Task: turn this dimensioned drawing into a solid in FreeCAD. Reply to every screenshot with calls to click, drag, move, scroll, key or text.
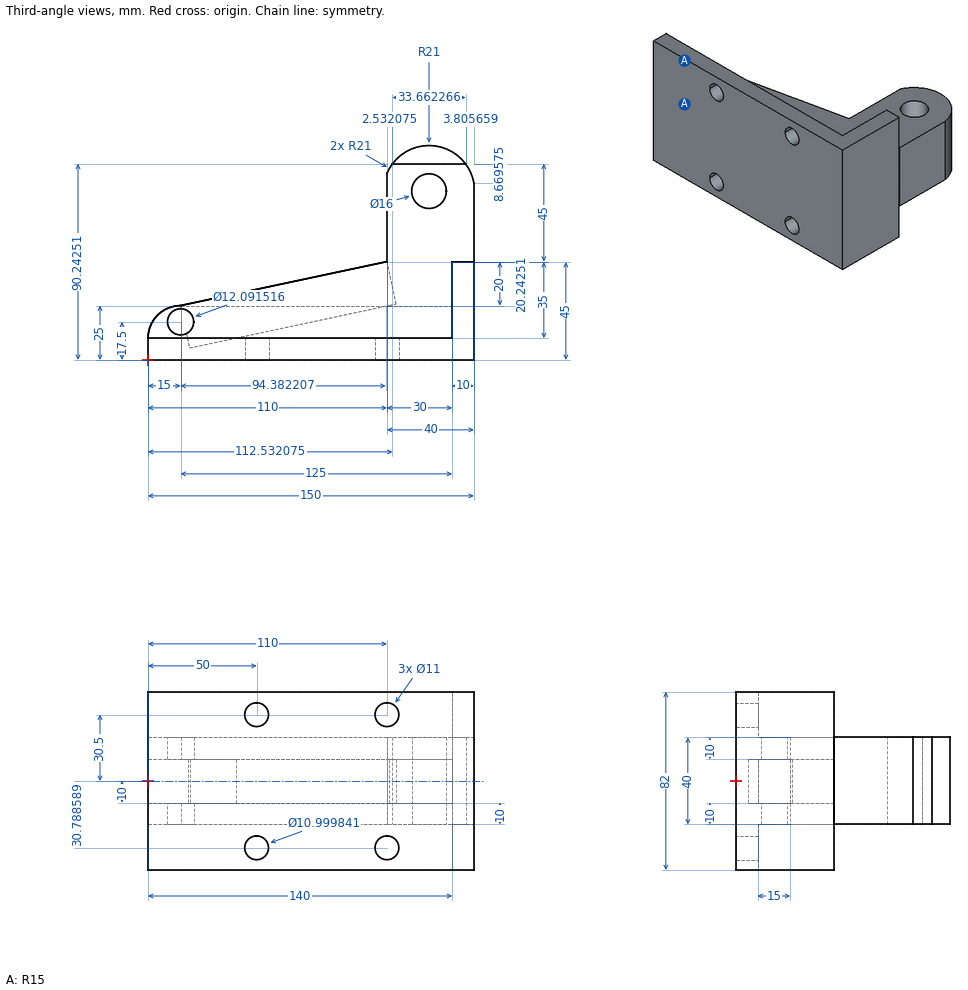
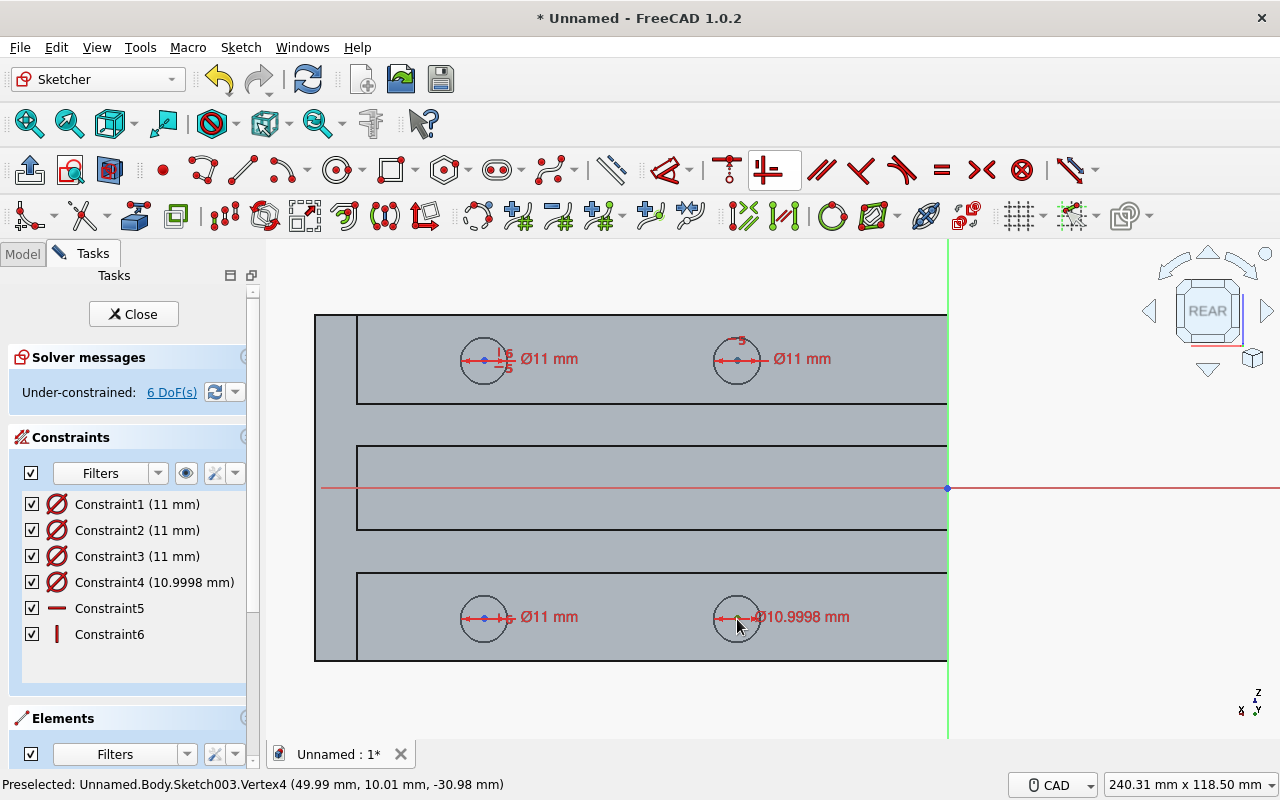
click(796, 170)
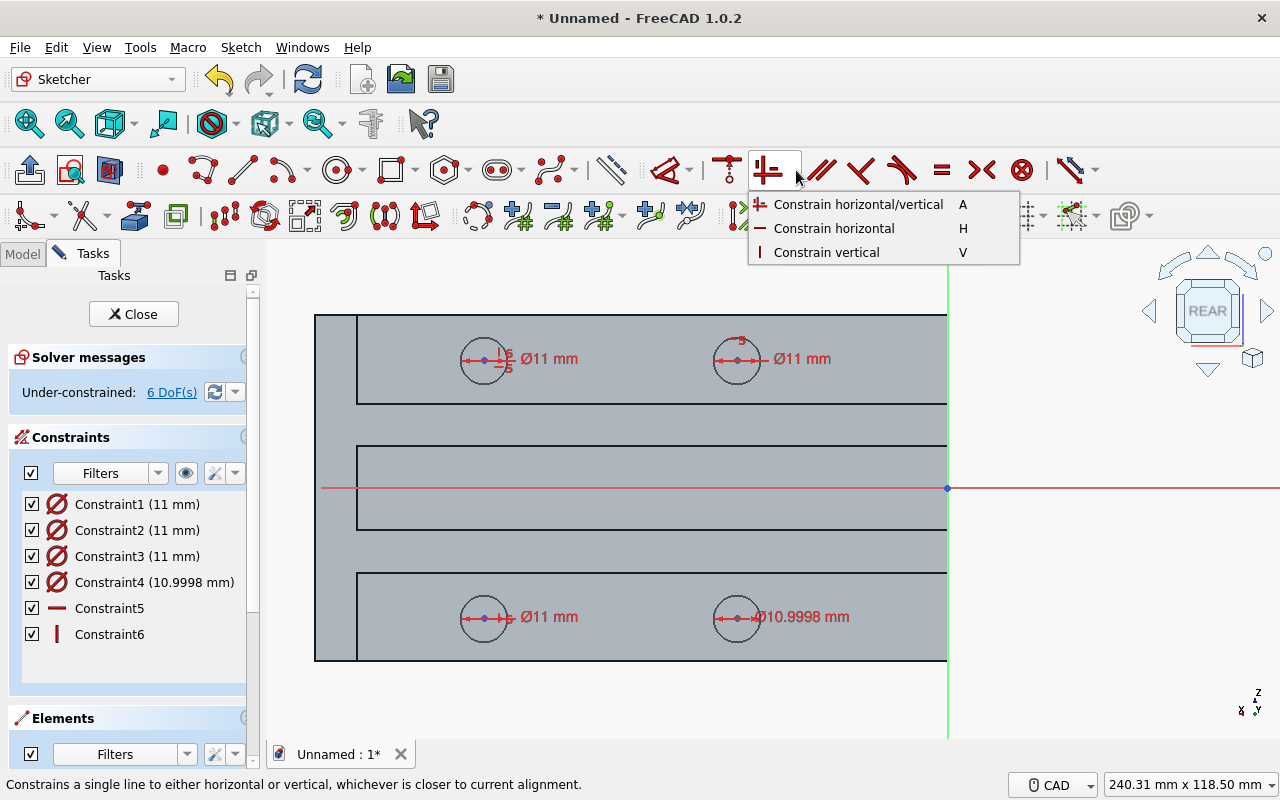
click(884, 252)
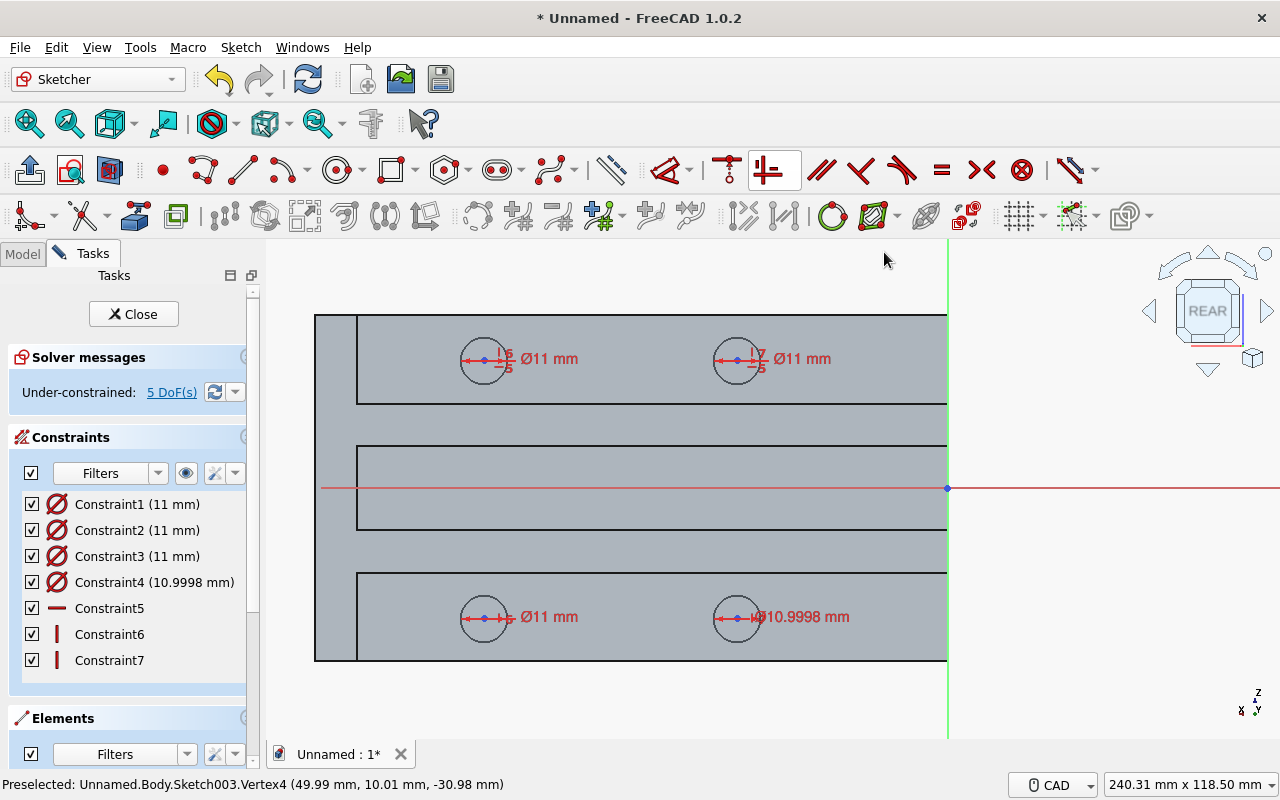
click(484, 619)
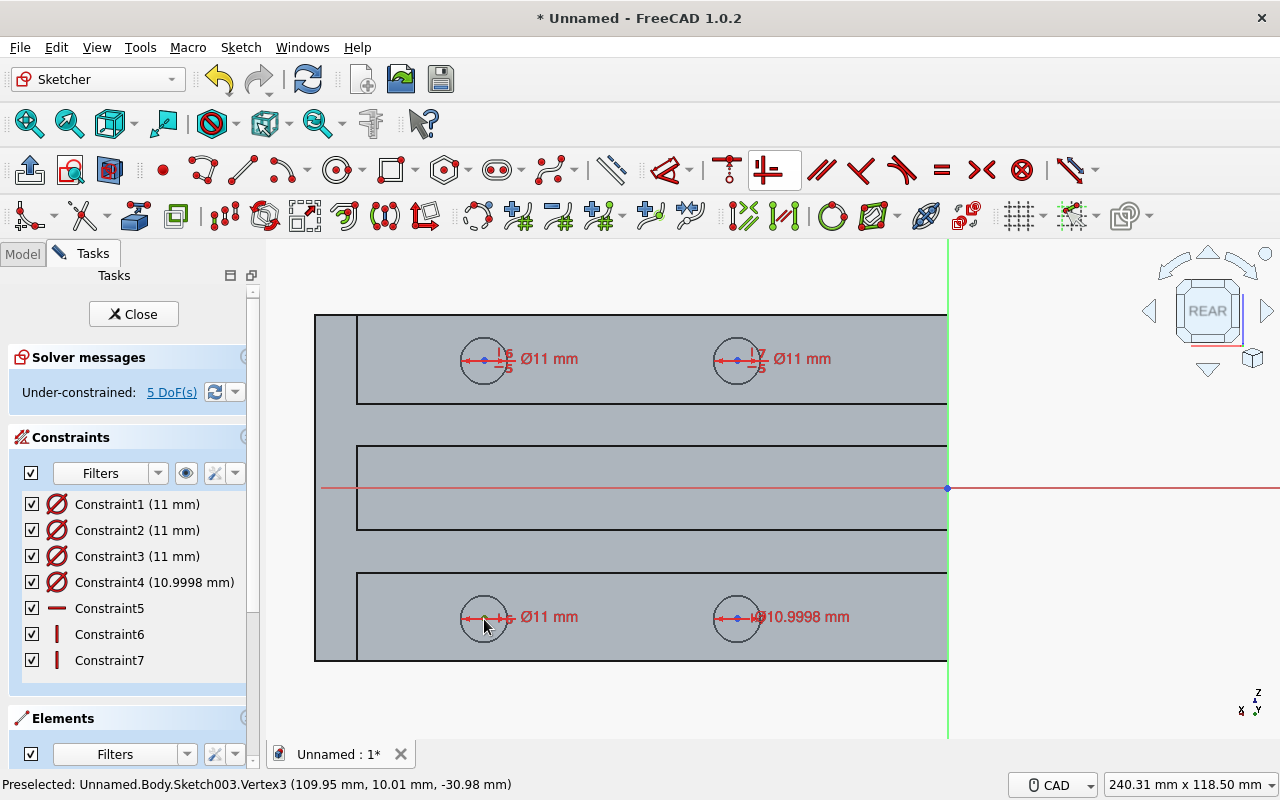
click(737, 619)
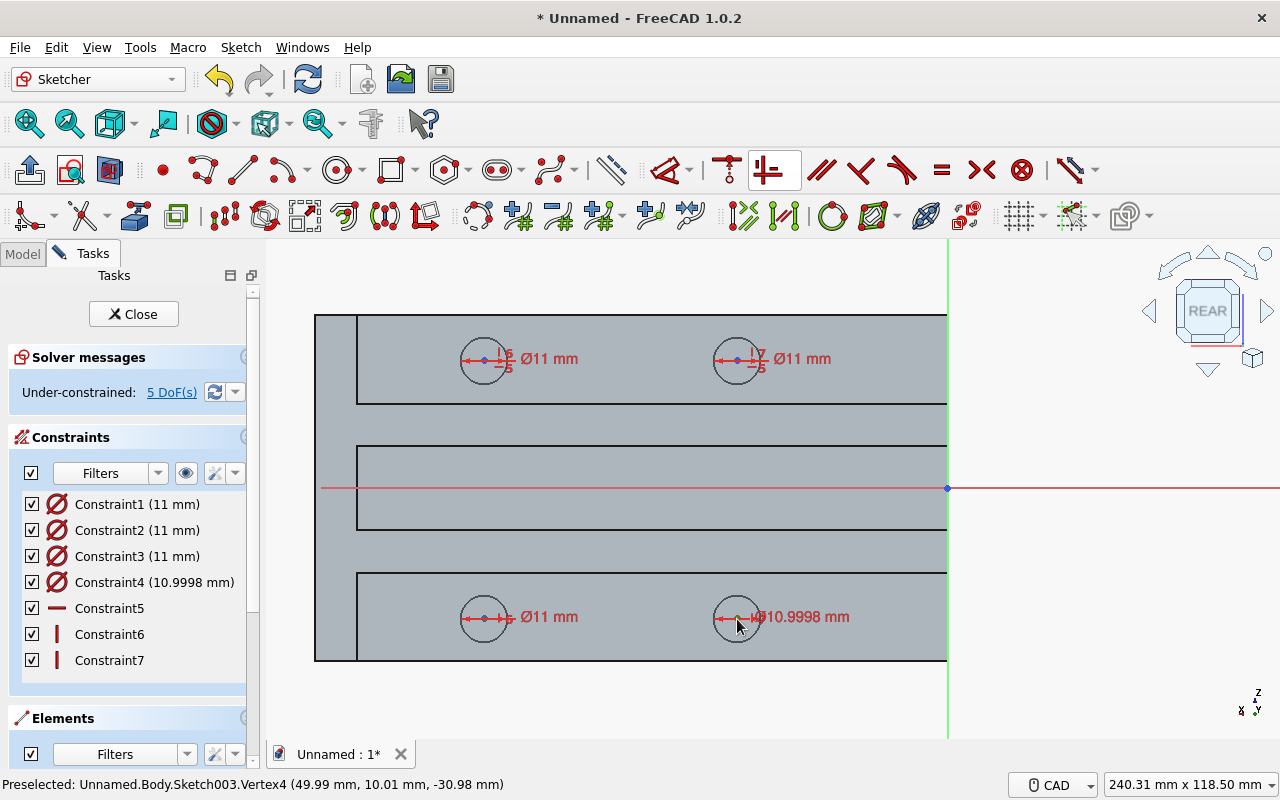
key(h)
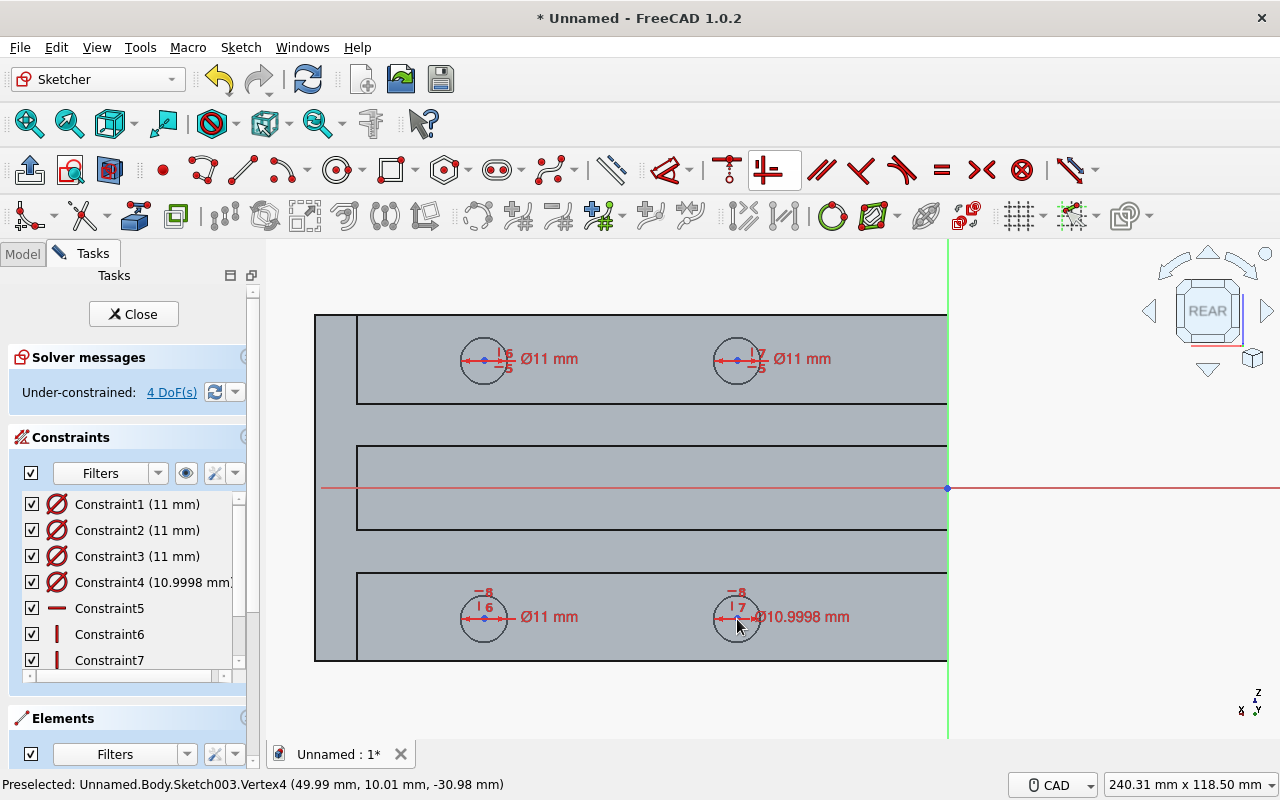
key(d)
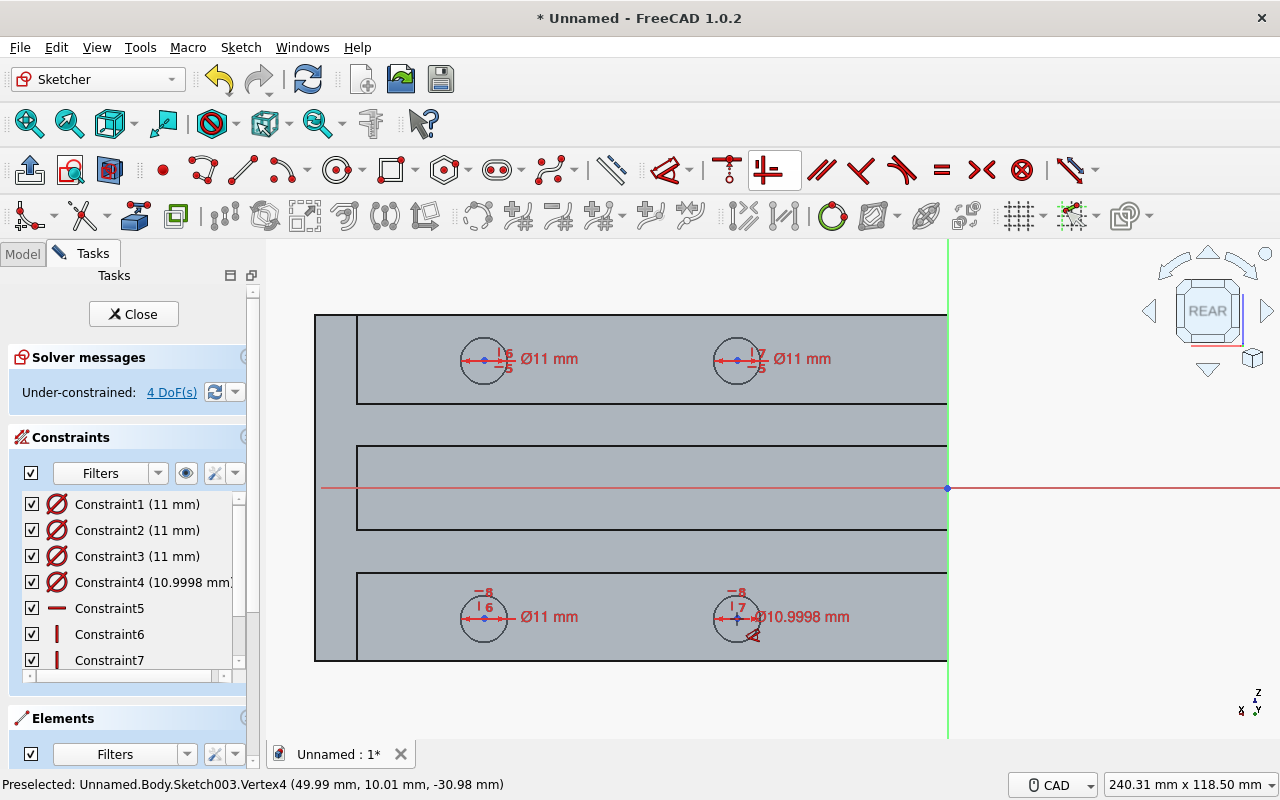
click(737, 361)
click(842, 327)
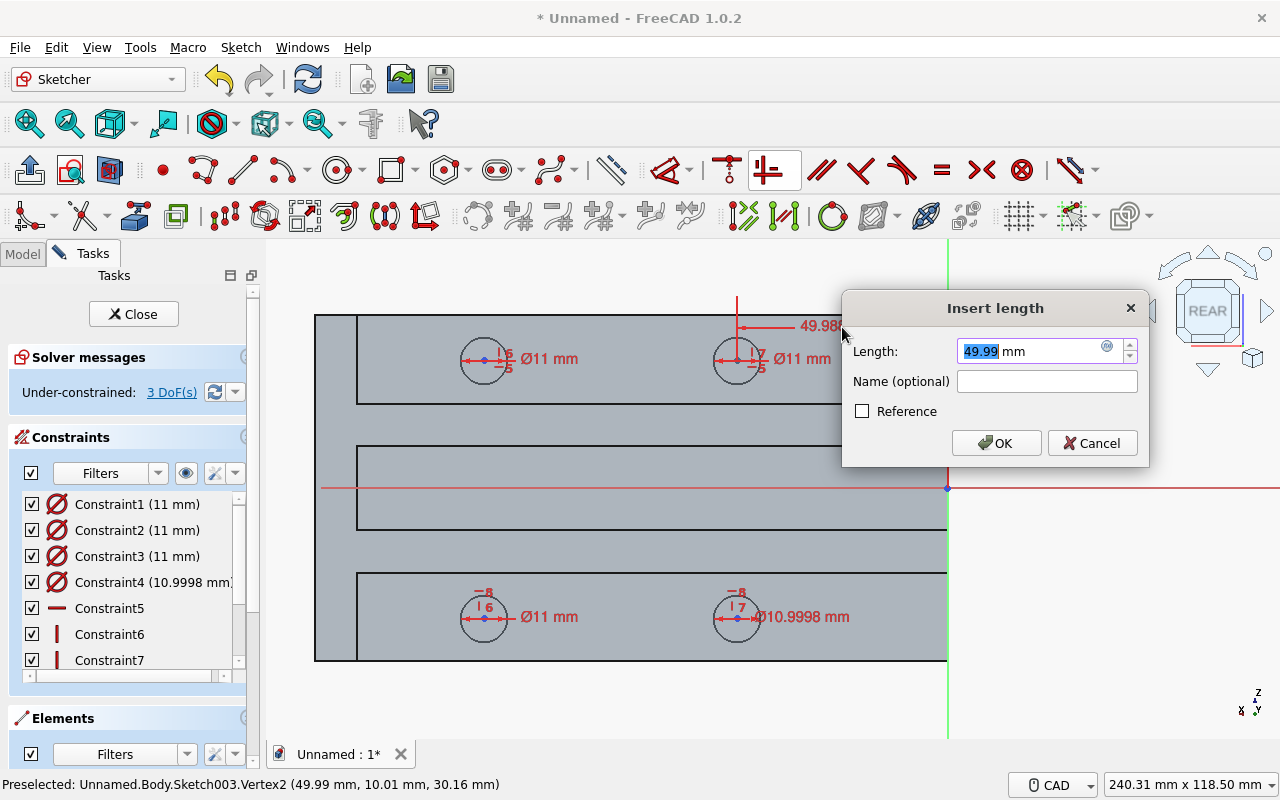
text(50)
key(Return)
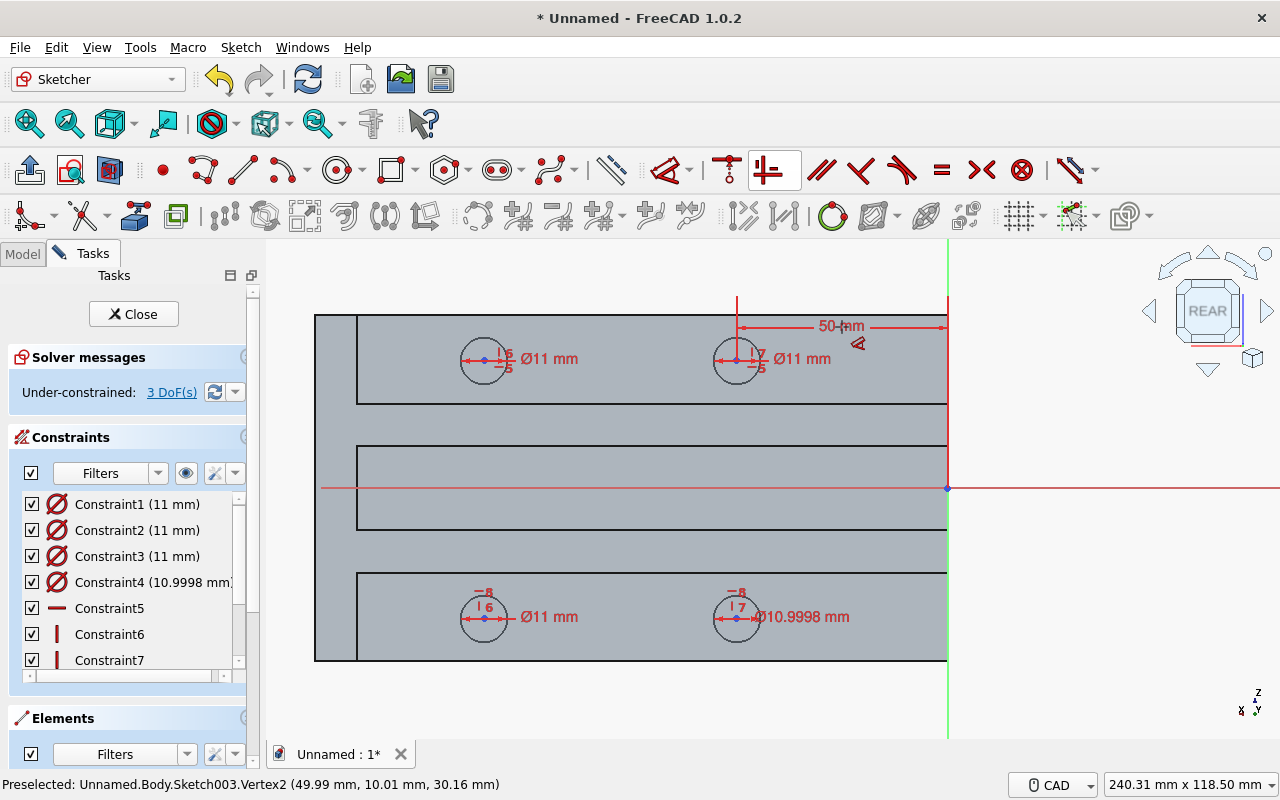
click(484, 361)
click(716, 327)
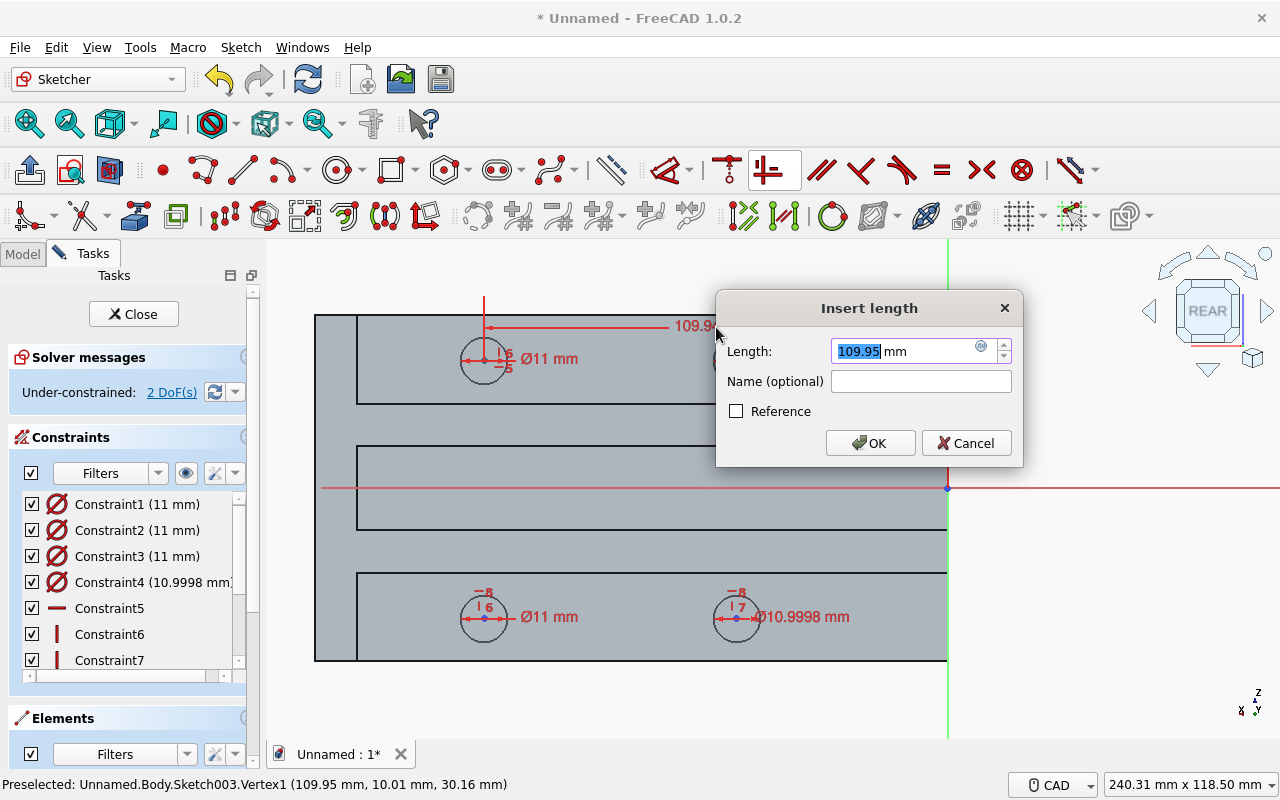
text(110)
key(Return)